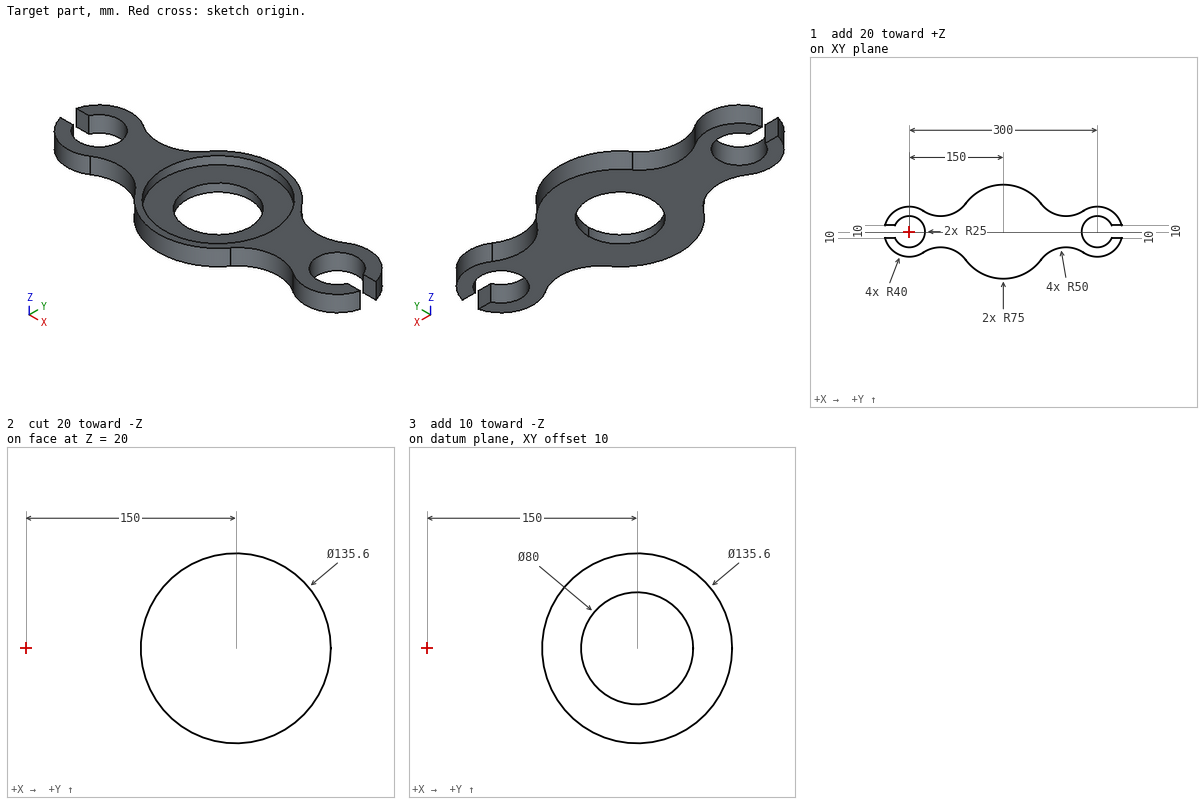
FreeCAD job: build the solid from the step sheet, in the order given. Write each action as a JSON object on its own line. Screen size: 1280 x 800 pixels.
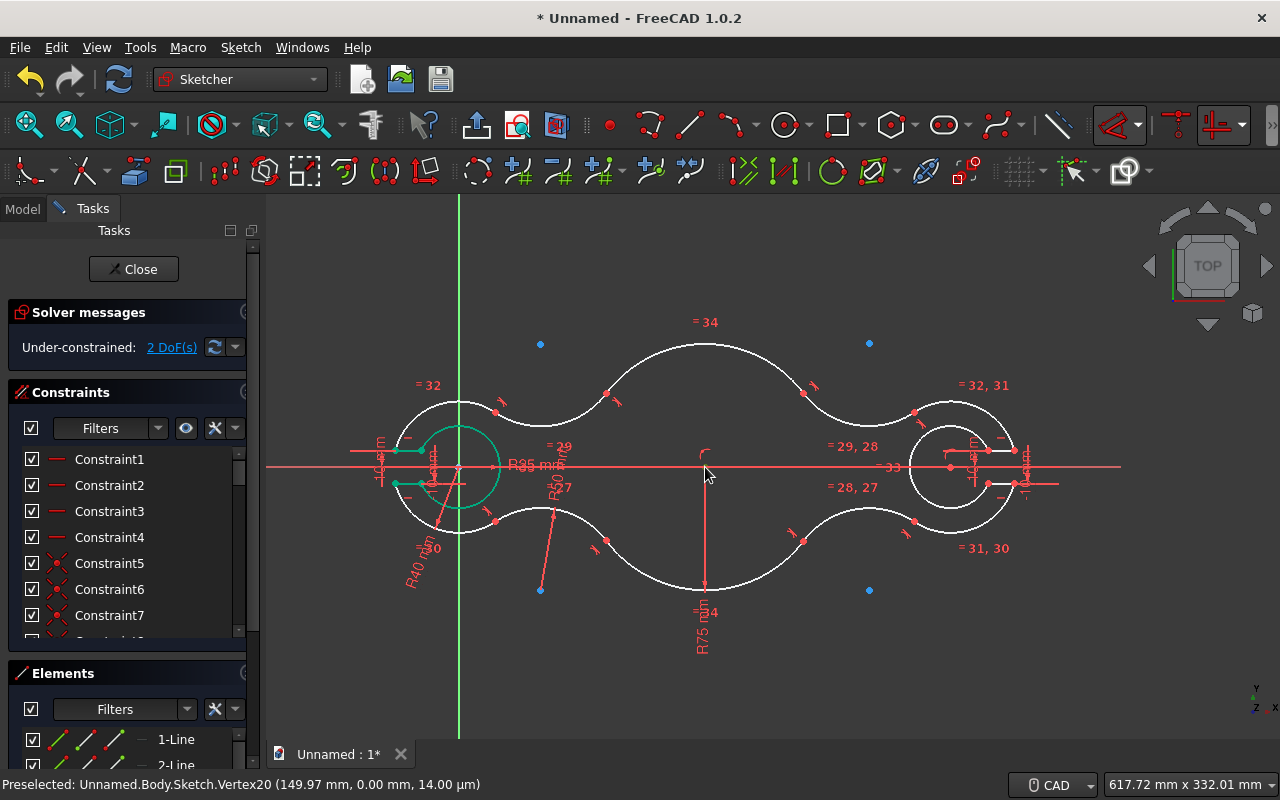
{"action": "left_click", "coordinate": [1140, 126]}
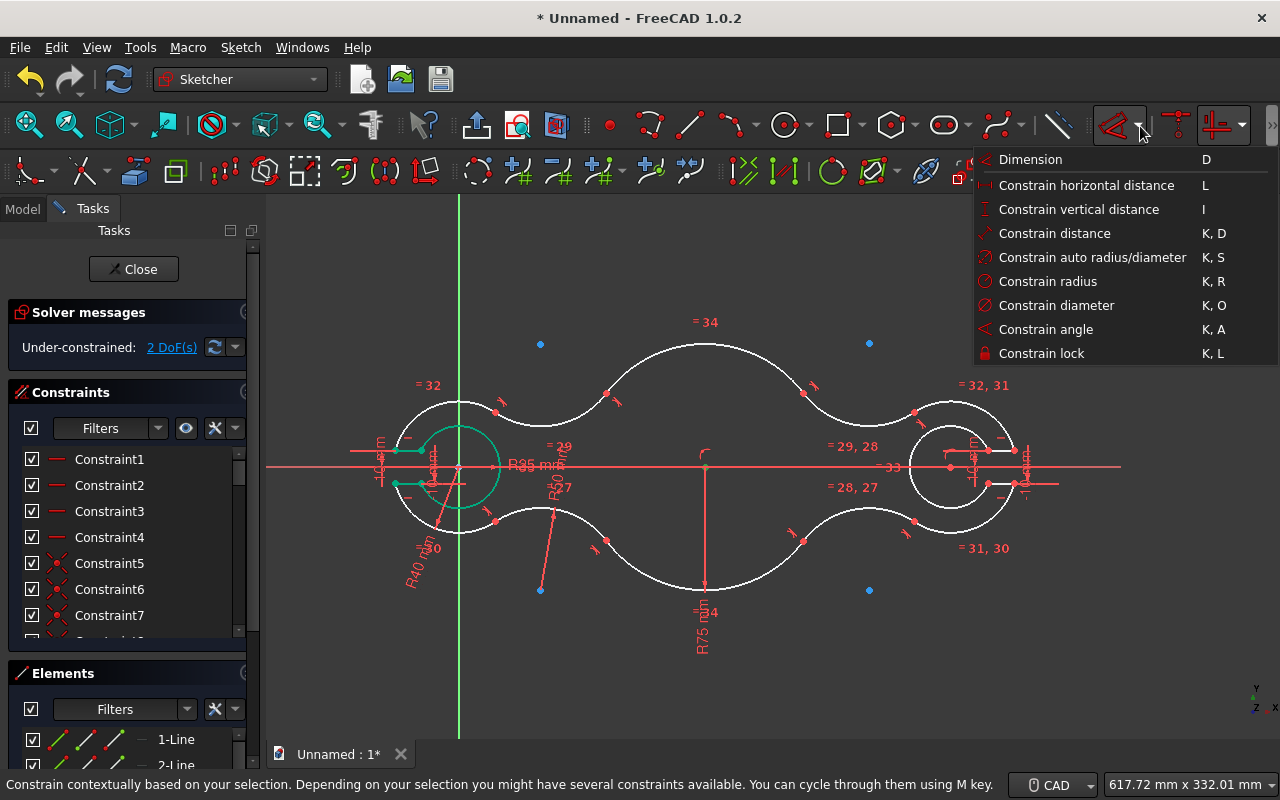
{"action": "left_click", "coordinate": [1126, 185]}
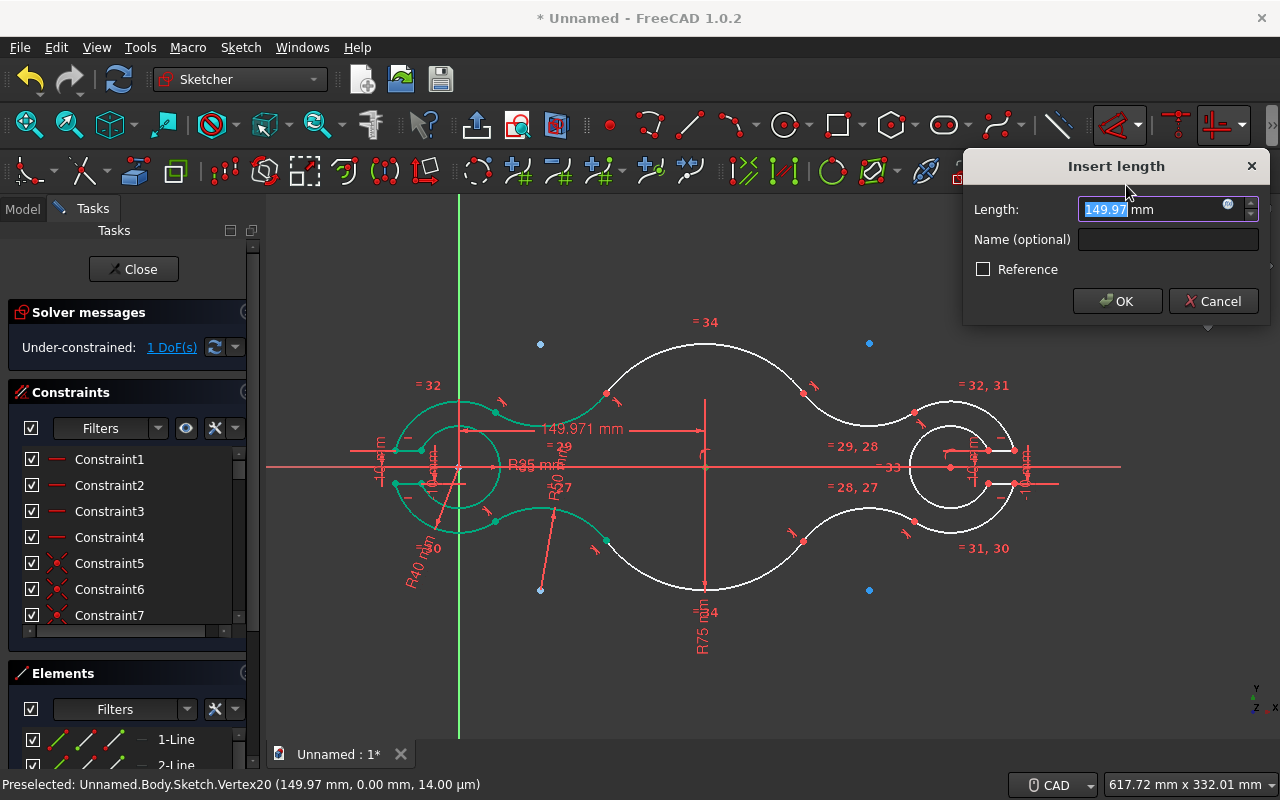
{"action": "type", "text": "150"}
{"action": "key", "text": "Return"}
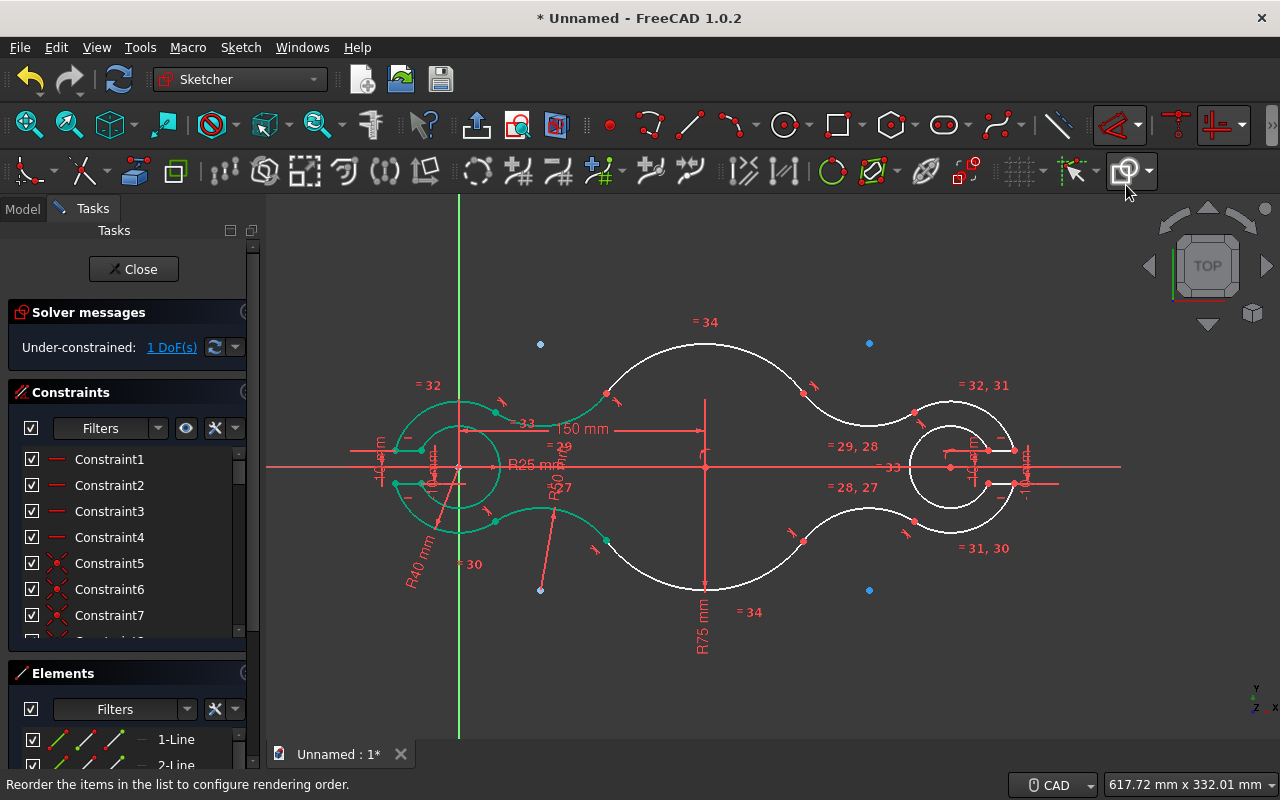
{"action": "left_click", "coordinate": [951, 467]}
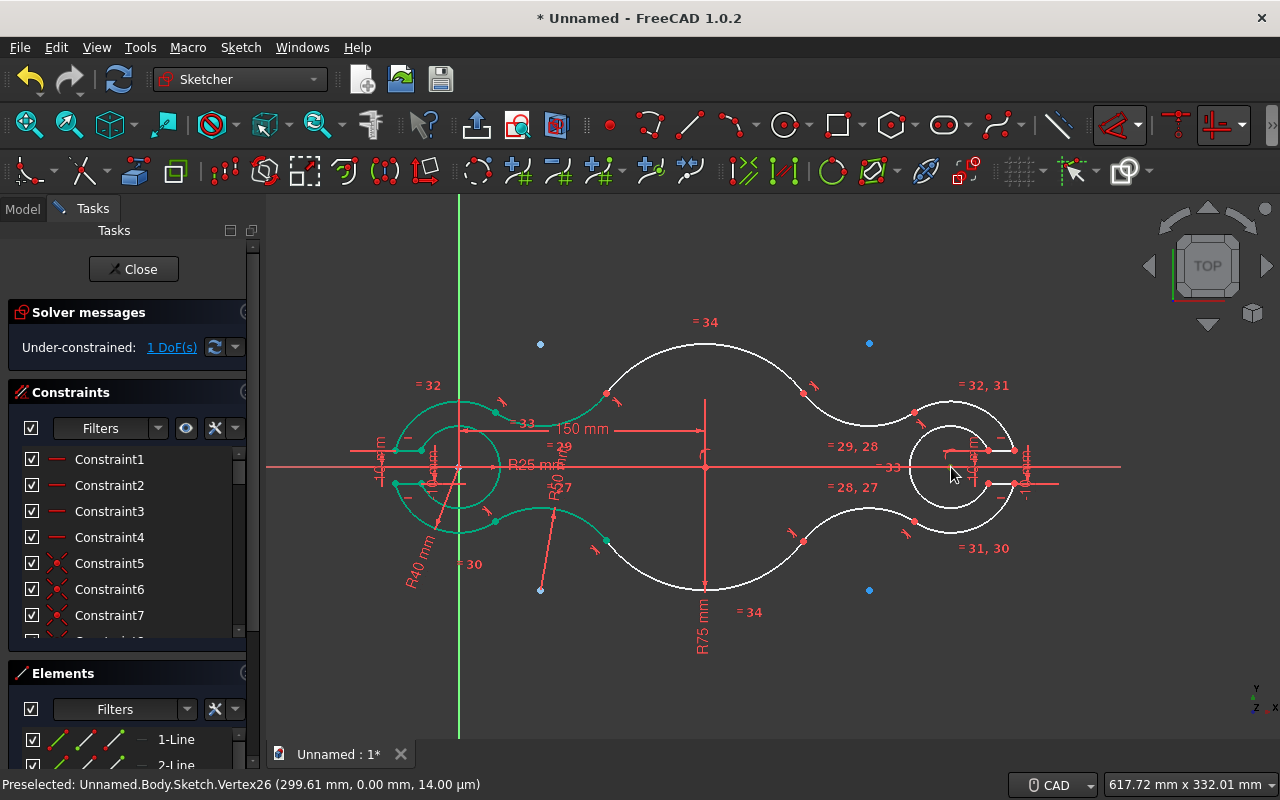
{"action": "key", "text": "l"}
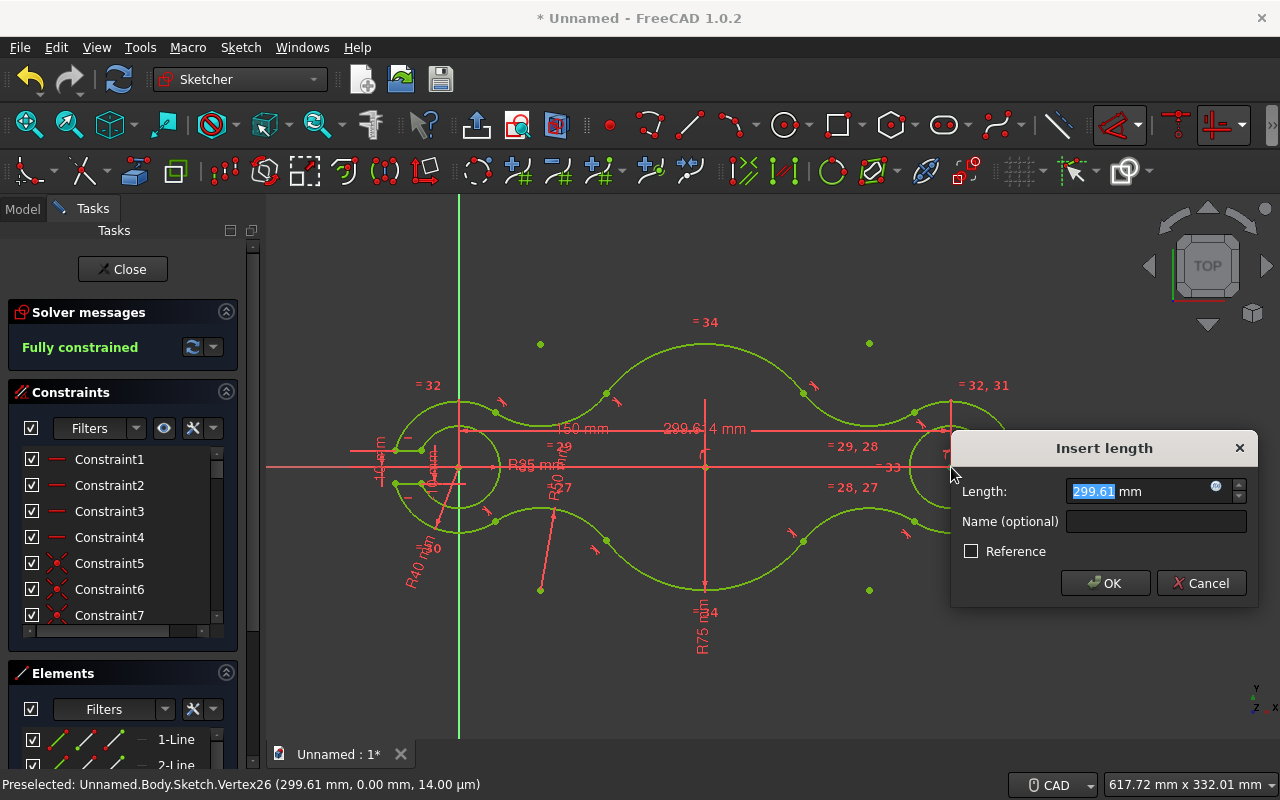
{"action": "type", "text": "300"}
{"action": "key", "text": "Return"}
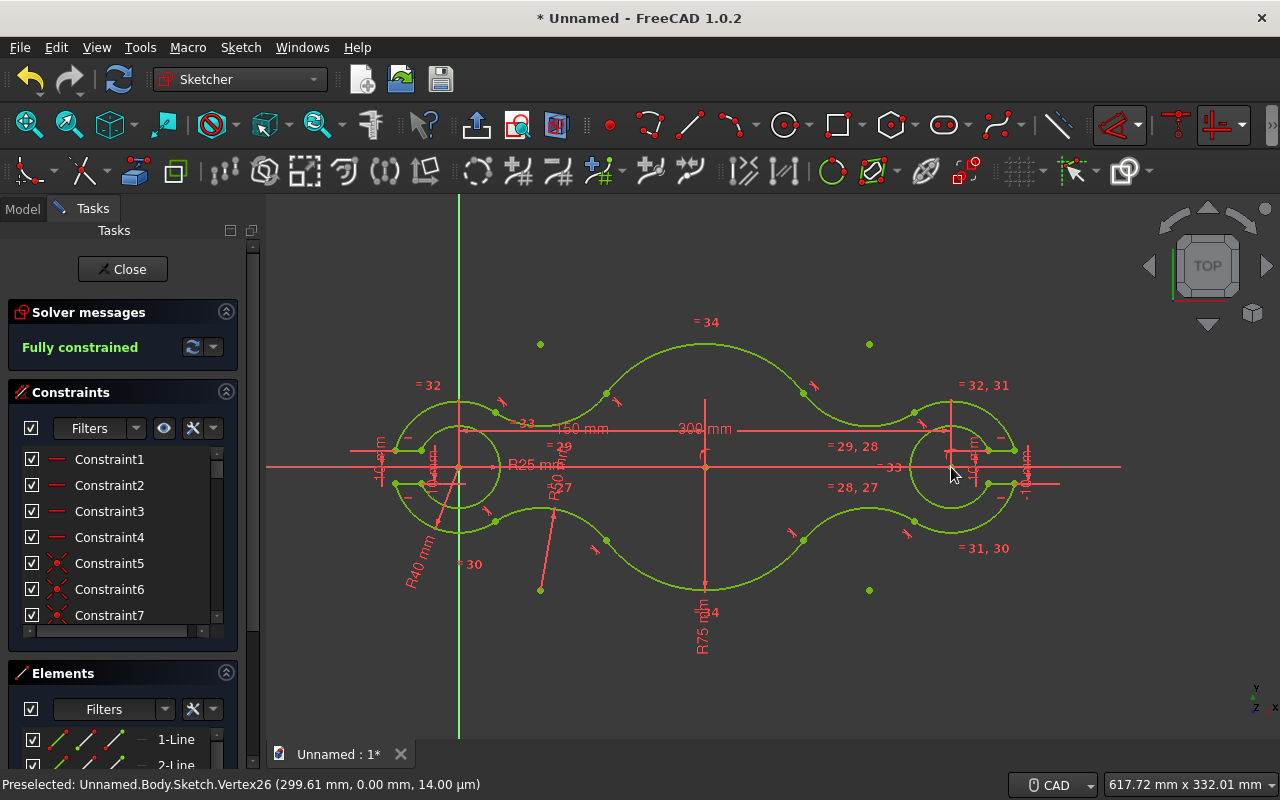
{"action": "left_click", "coordinate": [123, 269]}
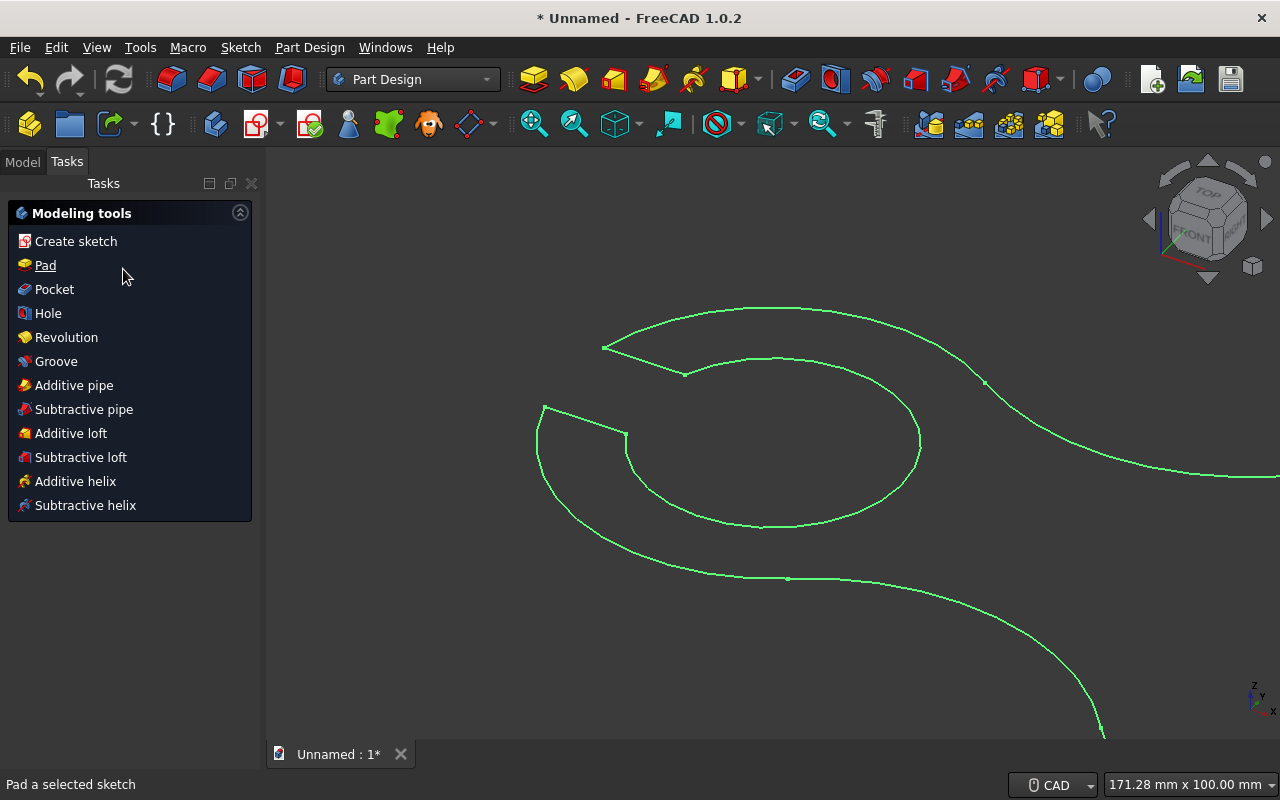
{"action": "left_click", "coordinate": [534, 80]}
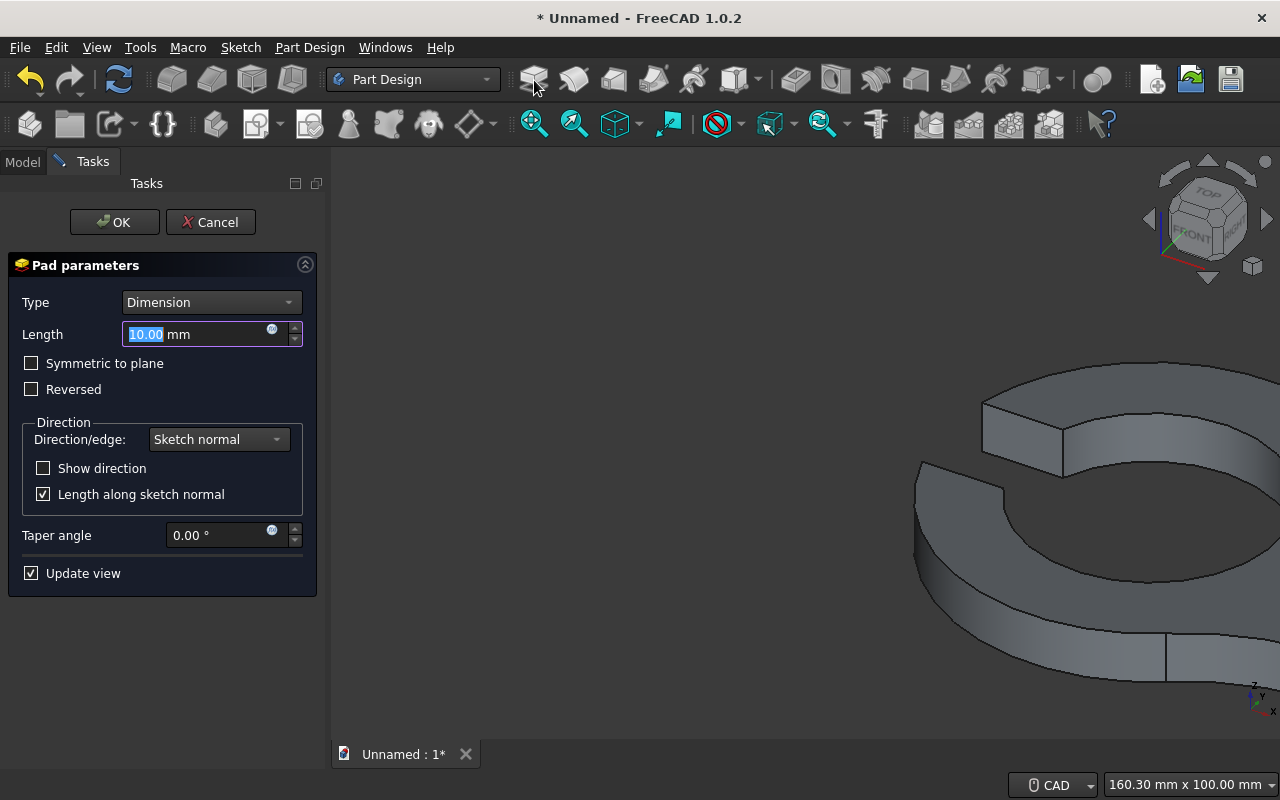
{"action": "type", "text": "20"}
{"action": "key", "text": "Tab"}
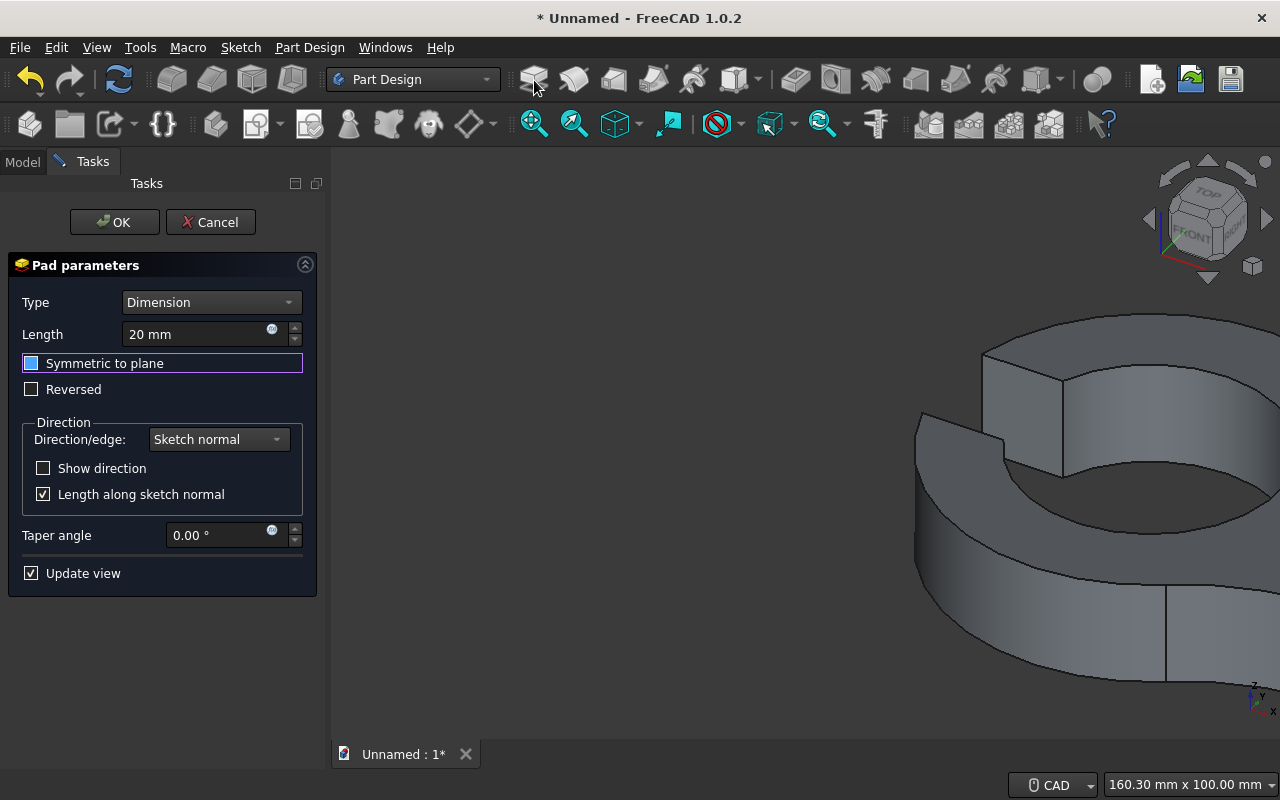
{"action": "left_click", "coordinate": [115, 222]}